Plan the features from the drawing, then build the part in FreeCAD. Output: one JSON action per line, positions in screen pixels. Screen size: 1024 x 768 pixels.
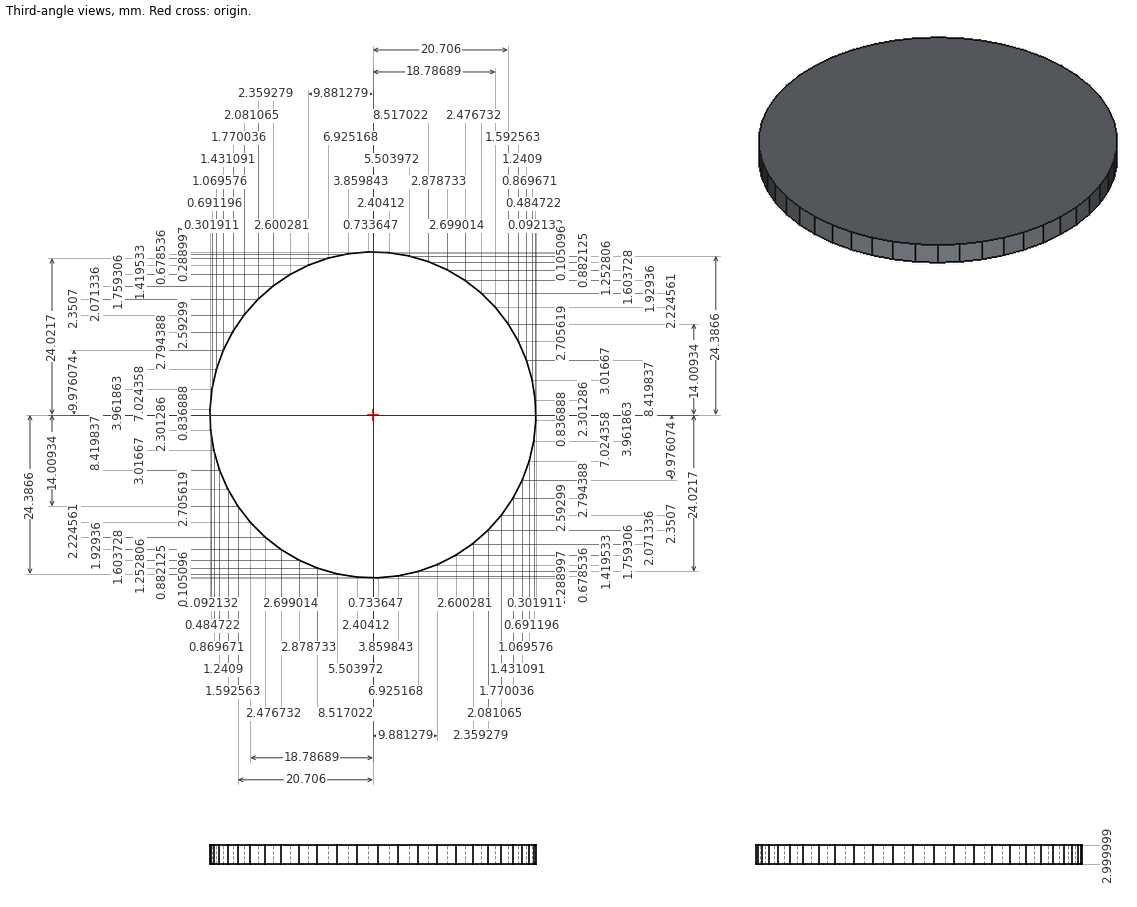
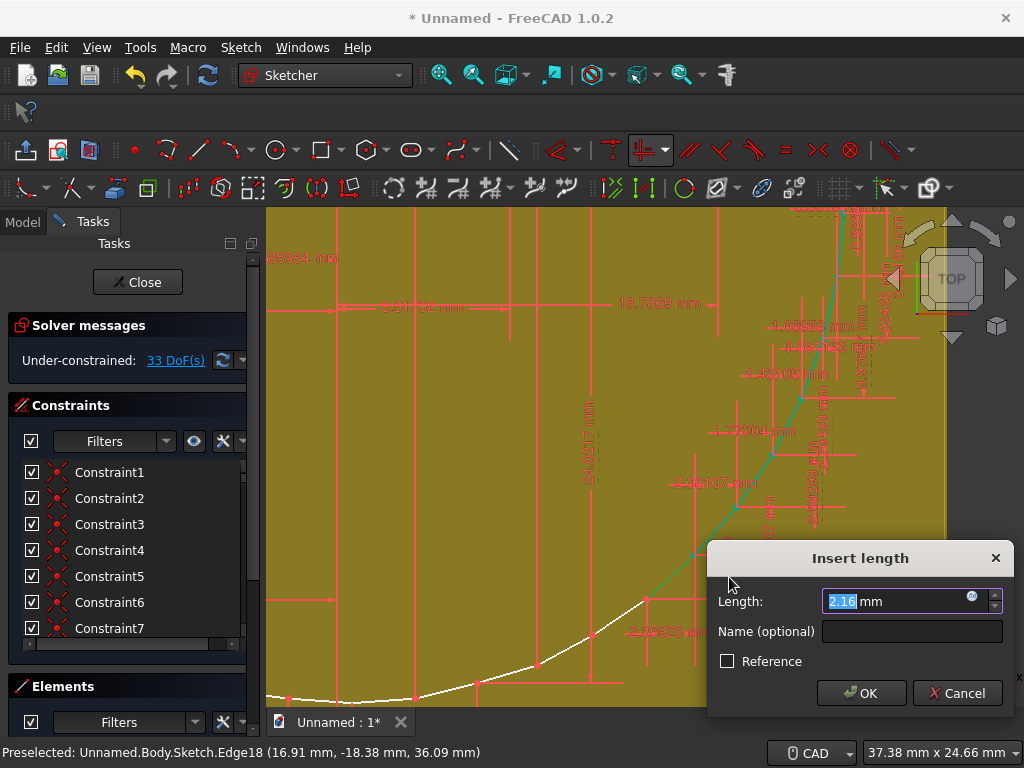
{"action": "type", "text": "2.071336"}
{"action": "key", "text": "Return"}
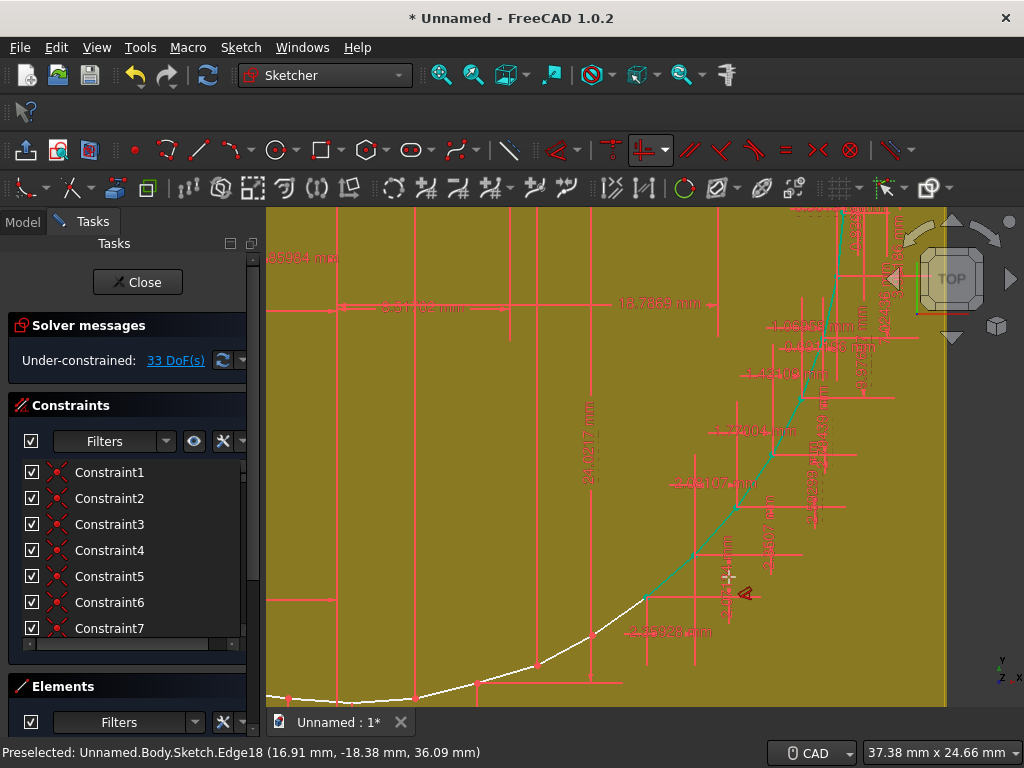
{"action": "left_click", "coordinate": [631, 609]}
{"action": "left_click", "coordinate": [620, 670]}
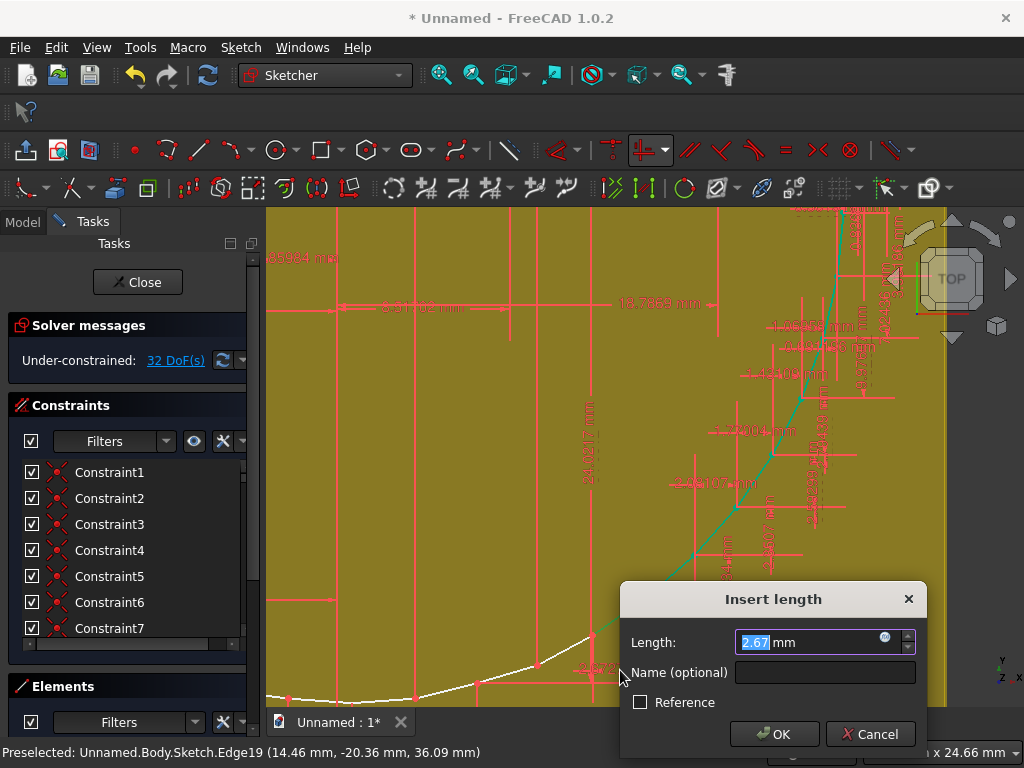
{"action": "type", "text": "2.600281"}
{"action": "key", "text": "Return"}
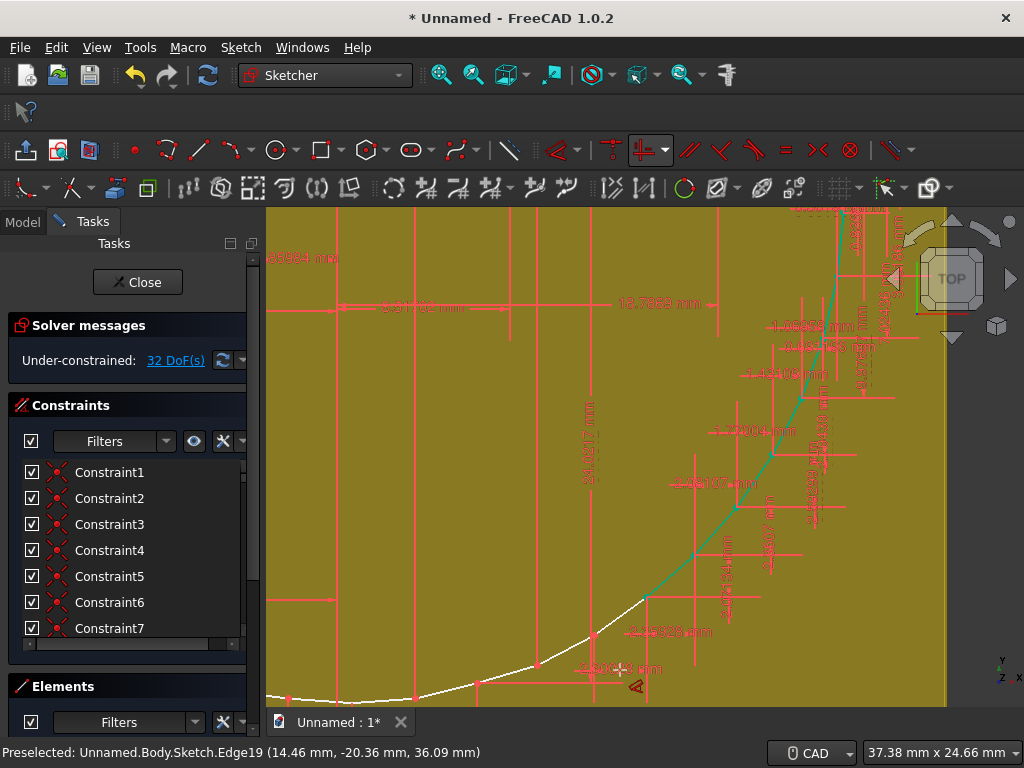
{"action": "left_click", "coordinate": [631, 609]}
{"action": "left_click", "coordinate": [681, 608]}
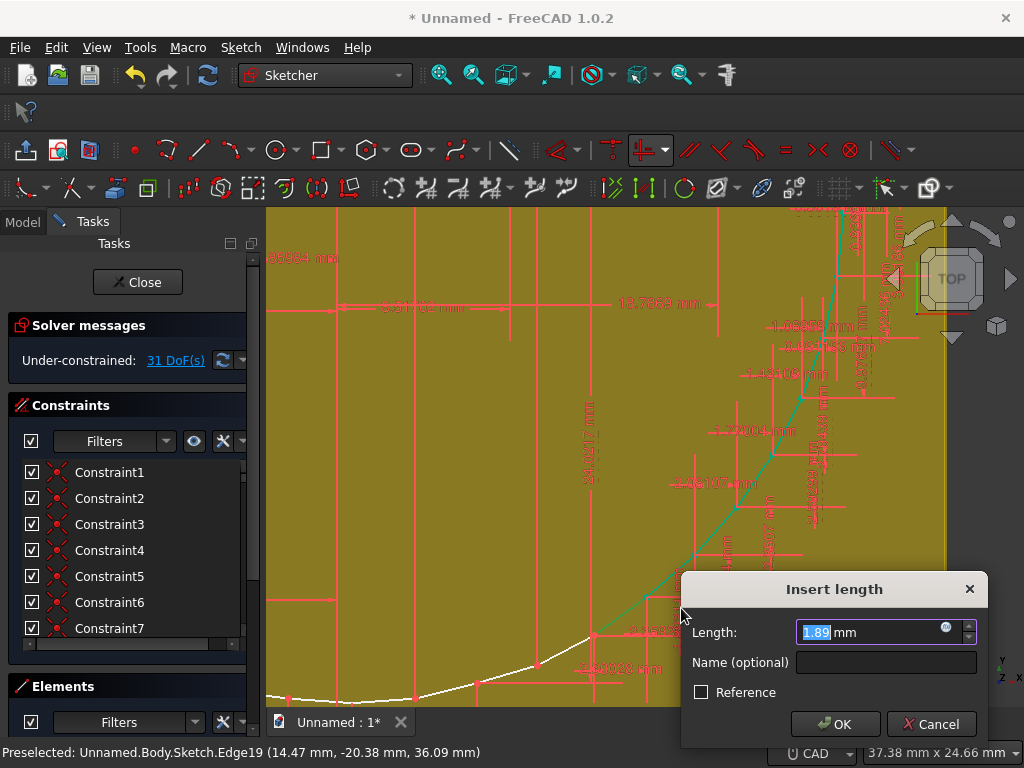
{"action": "type", "text": "1.759306"}
{"action": "key", "text": "Return"}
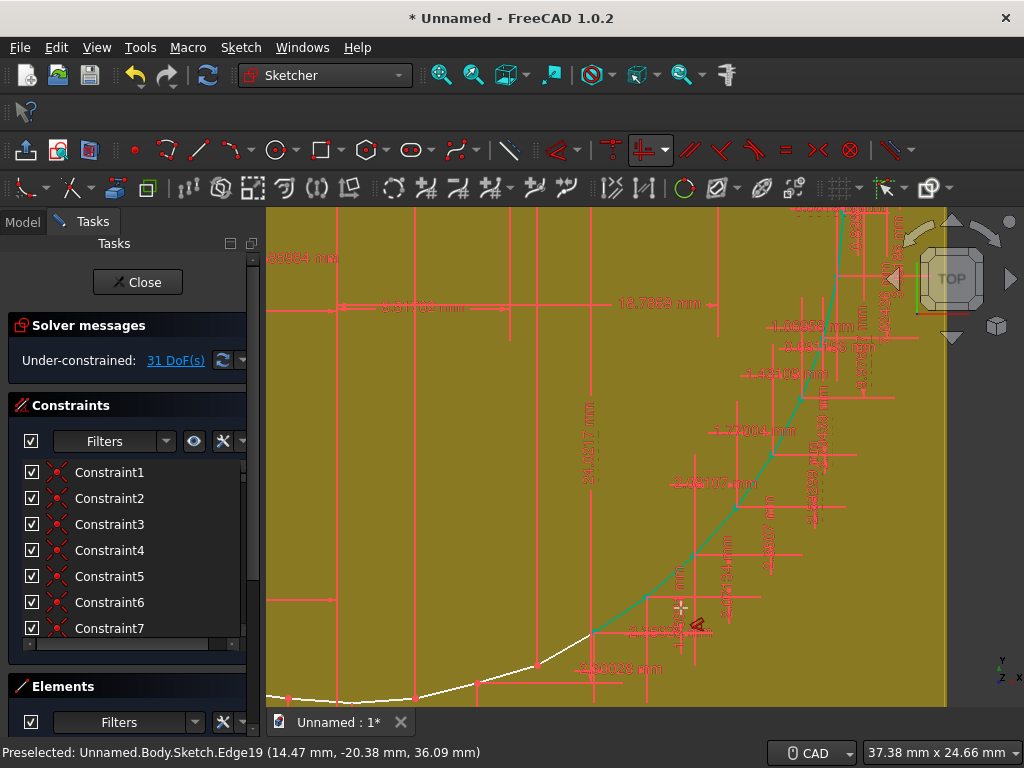
{"action": "scroll", "coordinate": [577, 643], "scroll_direction": "up", "scroll_amount": 2}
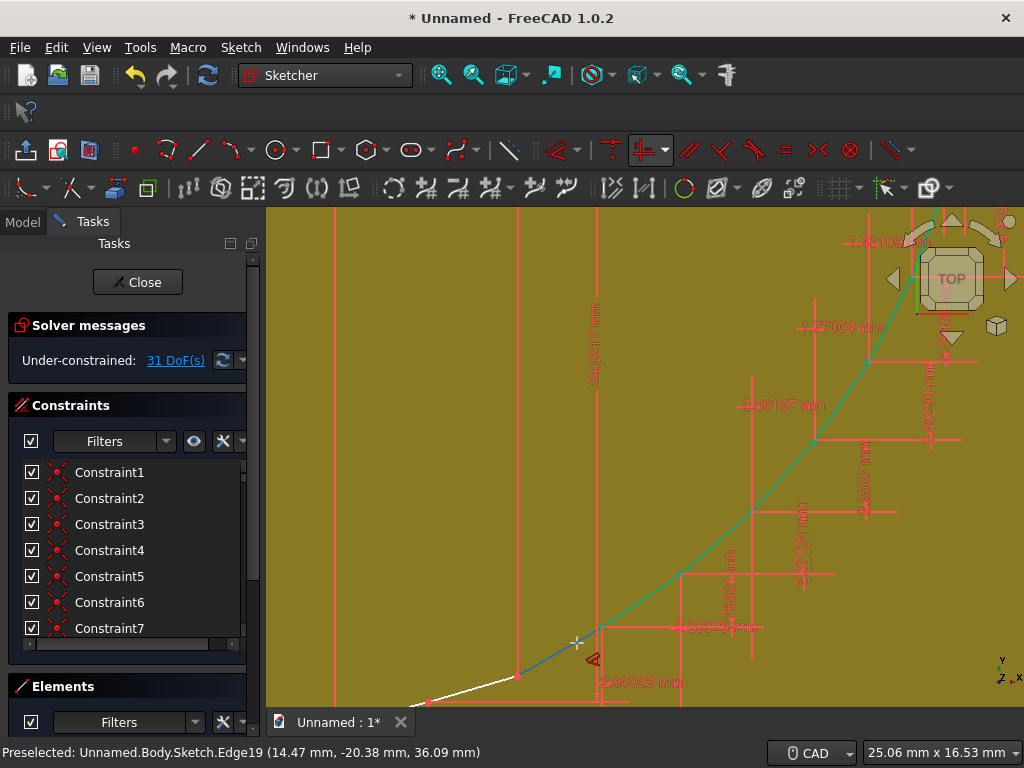
{"action": "left_click", "coordinate": [577, 642]}
{"action": "left_click", "coordinate": [636, 652]}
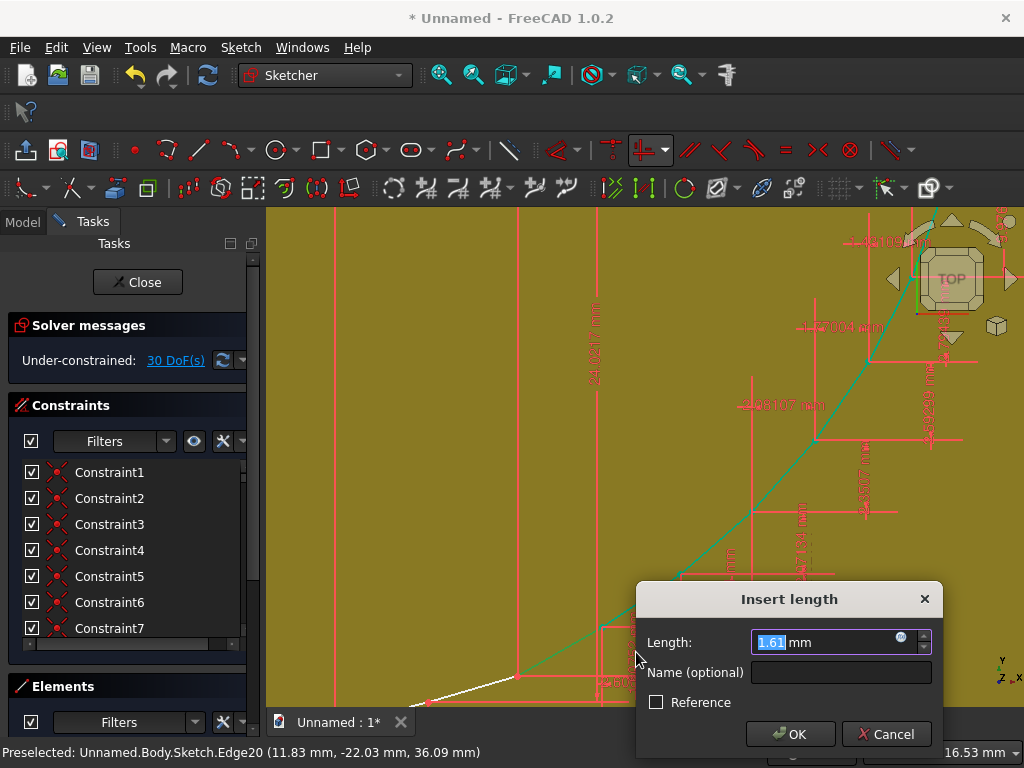
{"action": "type", "text": "1.419533"}
{"action": "key", "text": "Return"}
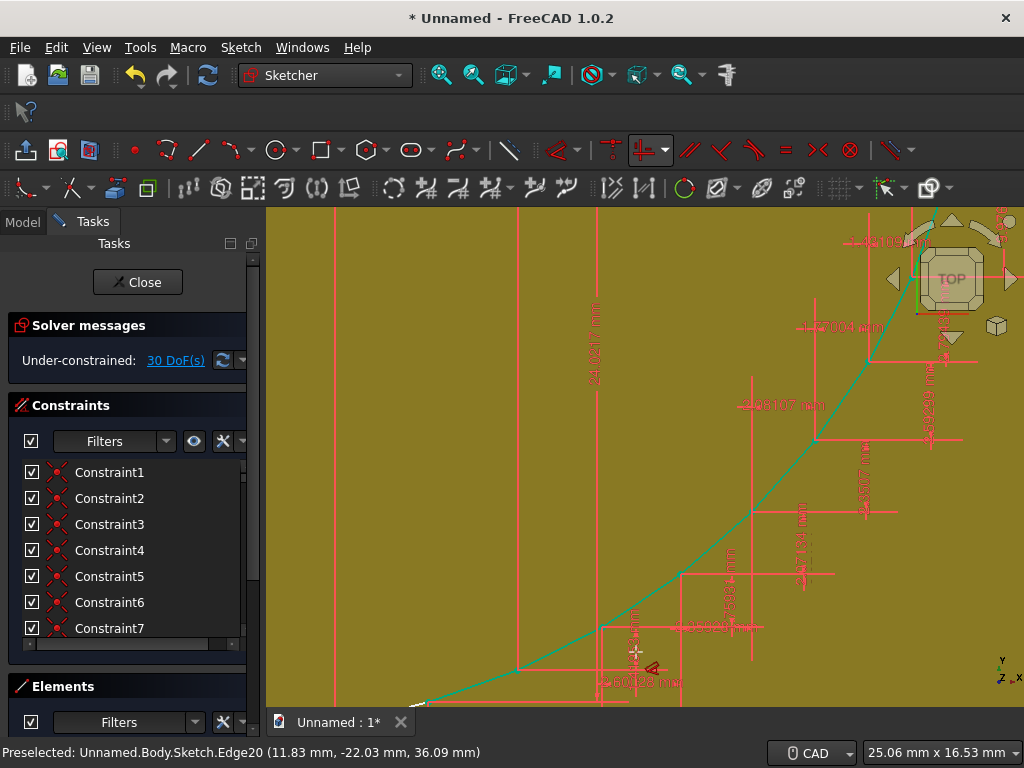
{"action": "scroll", "coordinate": [667, 579], "scroll_direction": "down", "scroll_amount": 8}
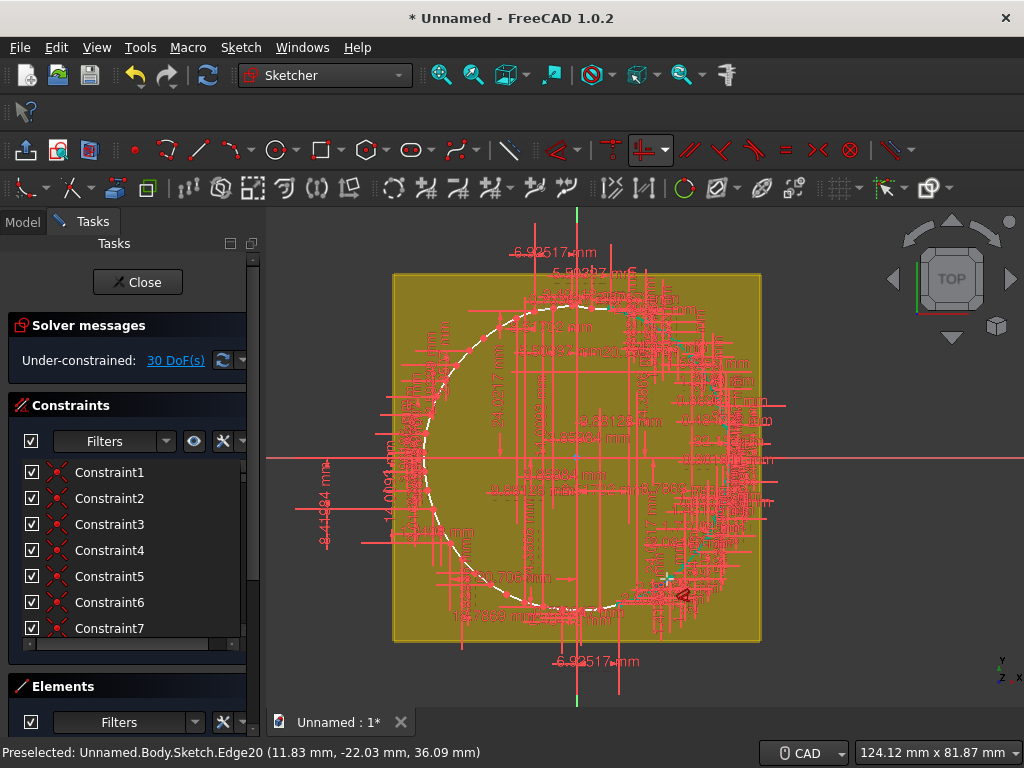
{"action": "scroll", "coordinate": [614, 606], "scroll_direction": "up", "scroll_amount": 12}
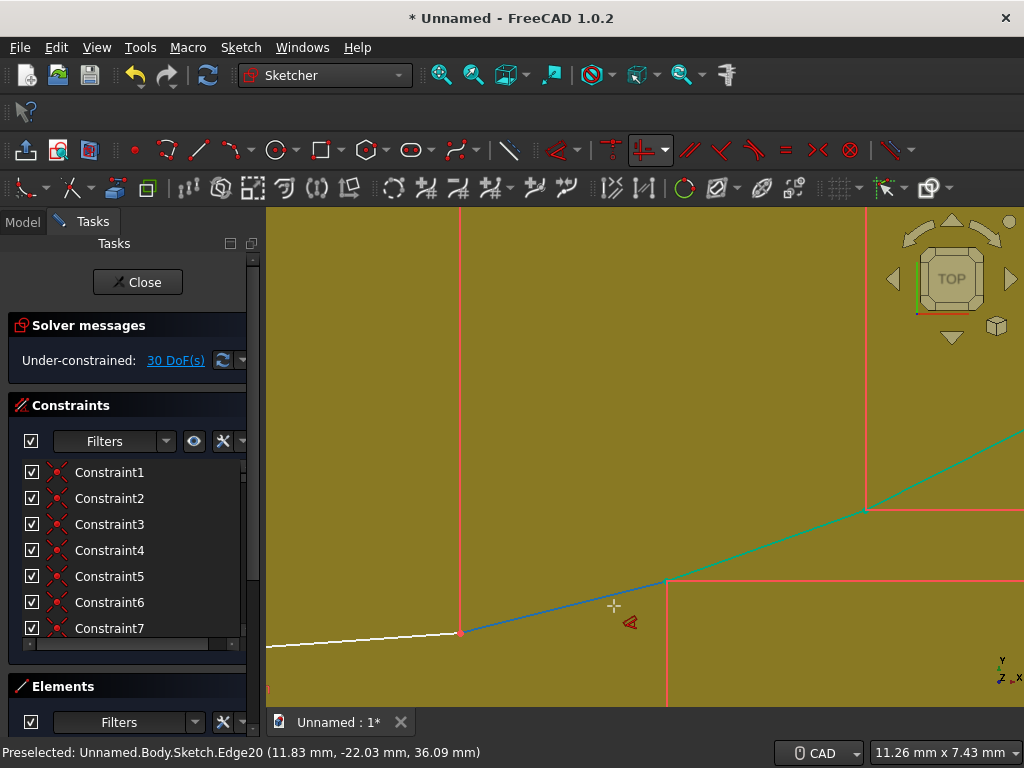
{"action": "left_click", "coordinate": [605, 597]}
{"action": "left_click", "coordinate": [701, 607]}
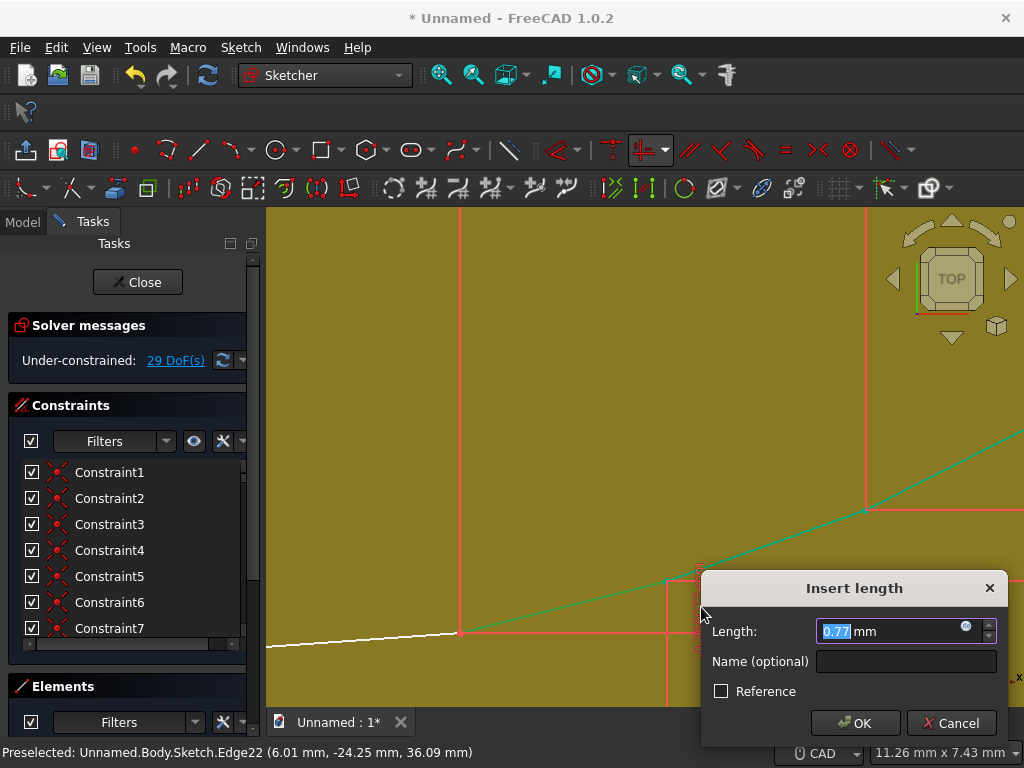
{"action": "type", "text": "0.678536"}
{"action": "key", "text": "Return"}